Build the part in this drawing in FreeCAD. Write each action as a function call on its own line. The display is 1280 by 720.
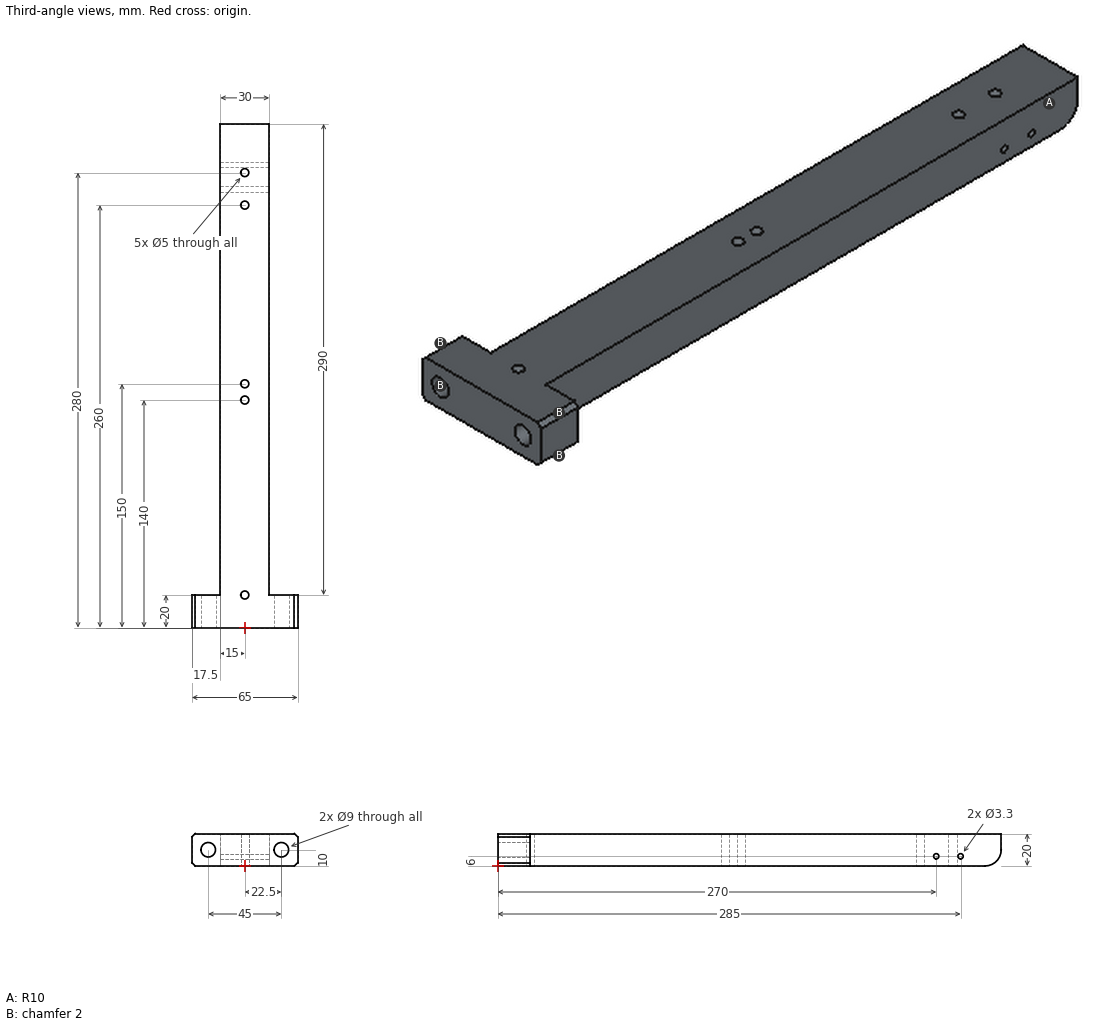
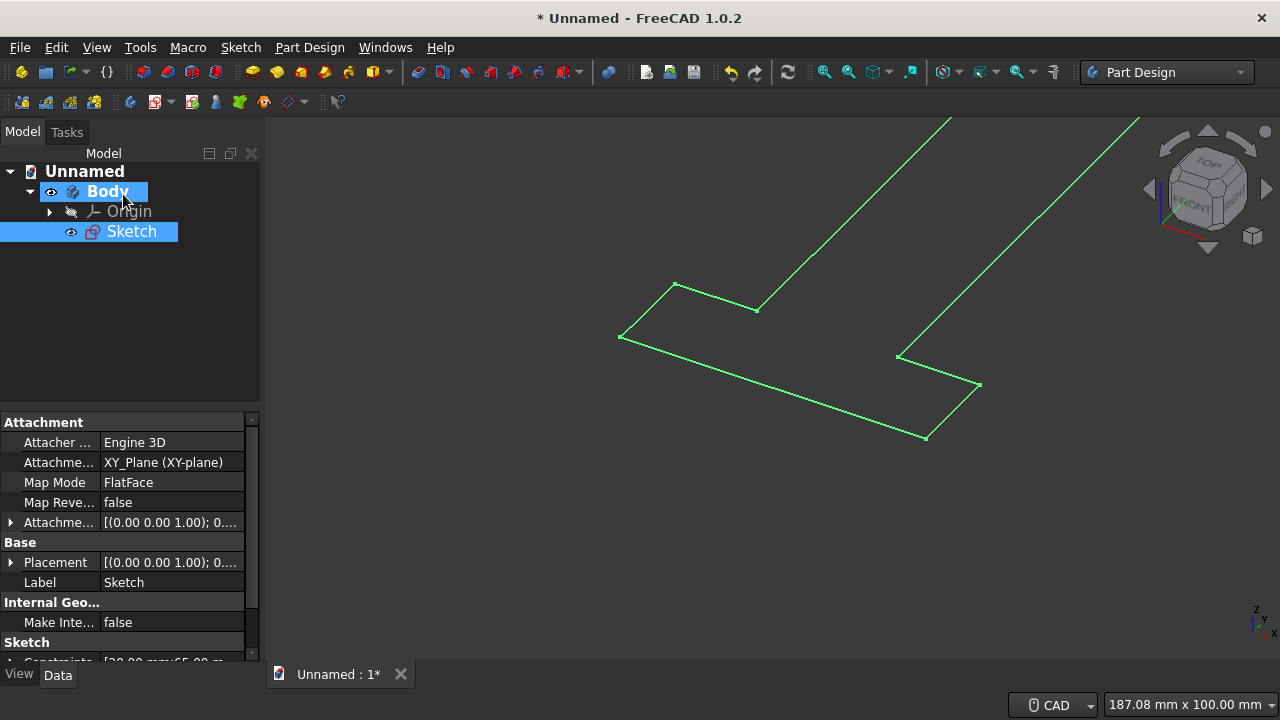
click(254, 72)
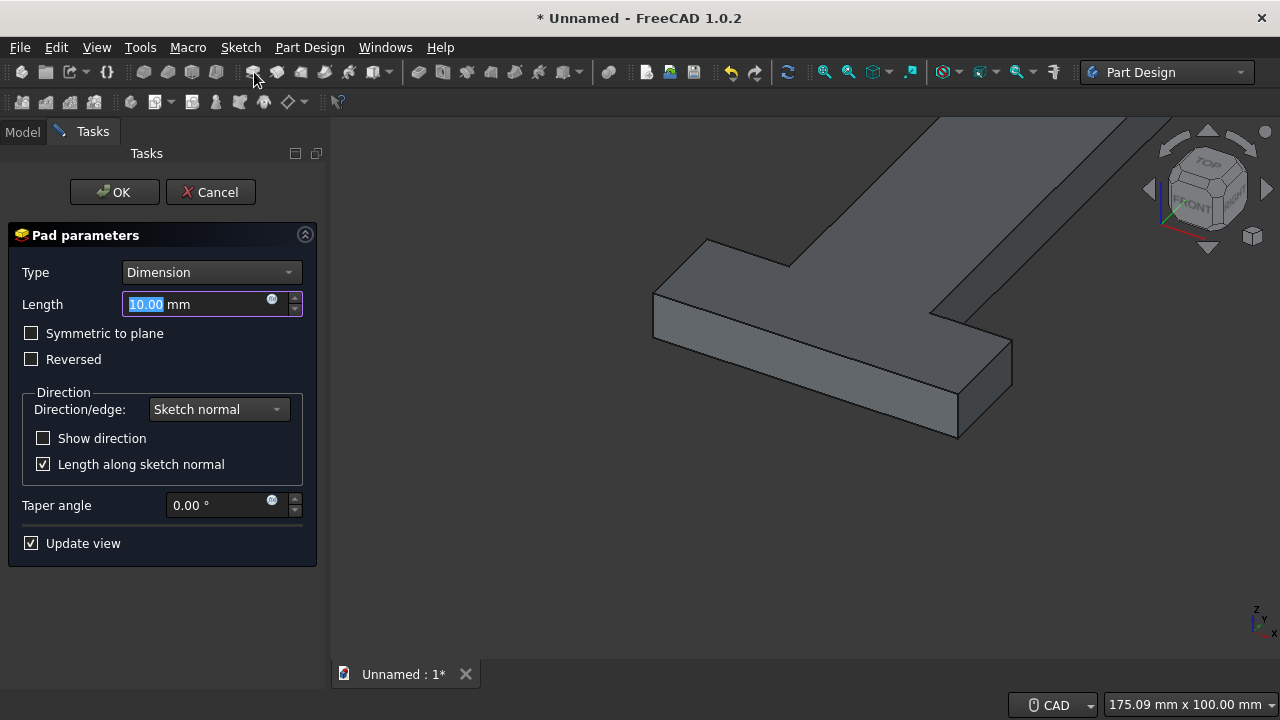
text(20)
key(Tab)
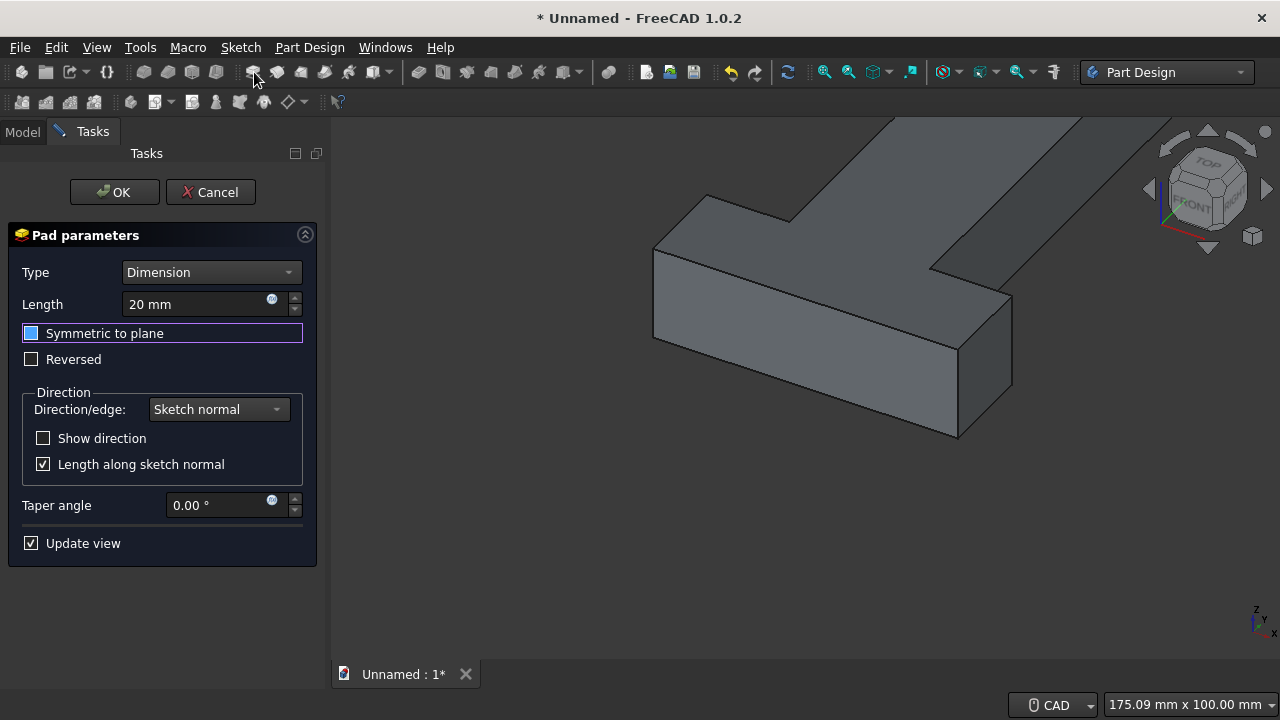
click(115, 192)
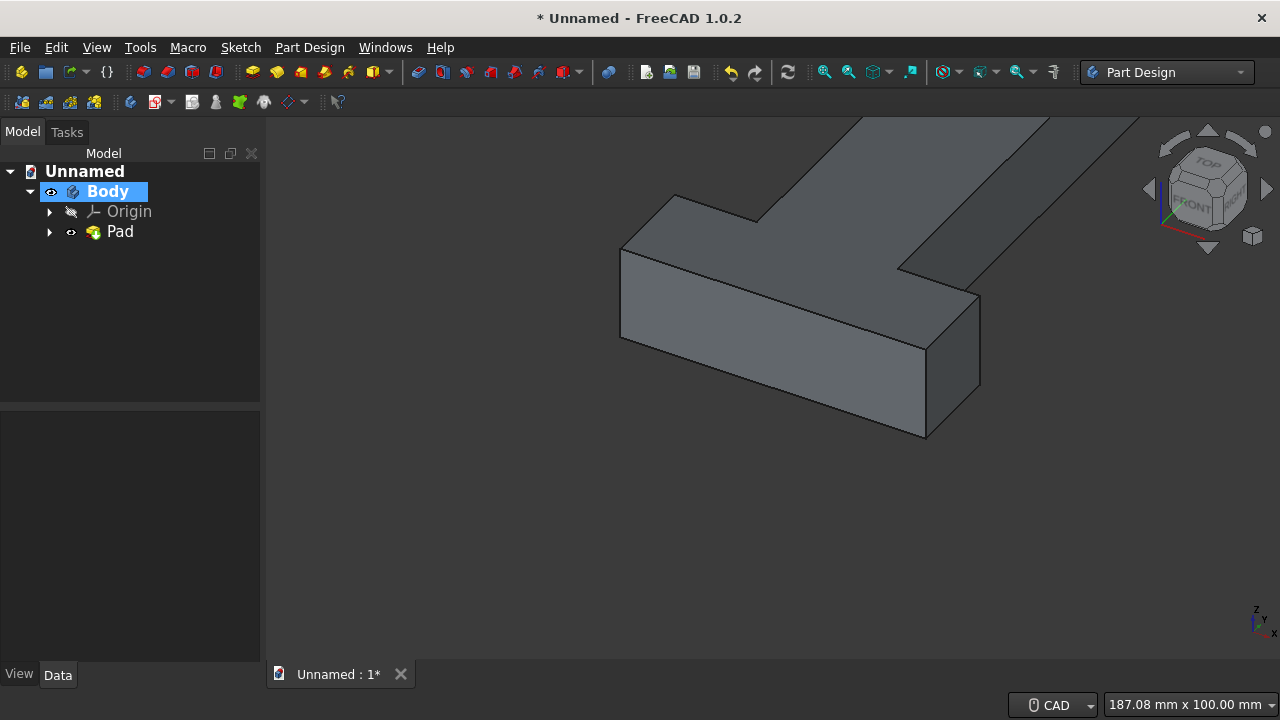
click(826, 72)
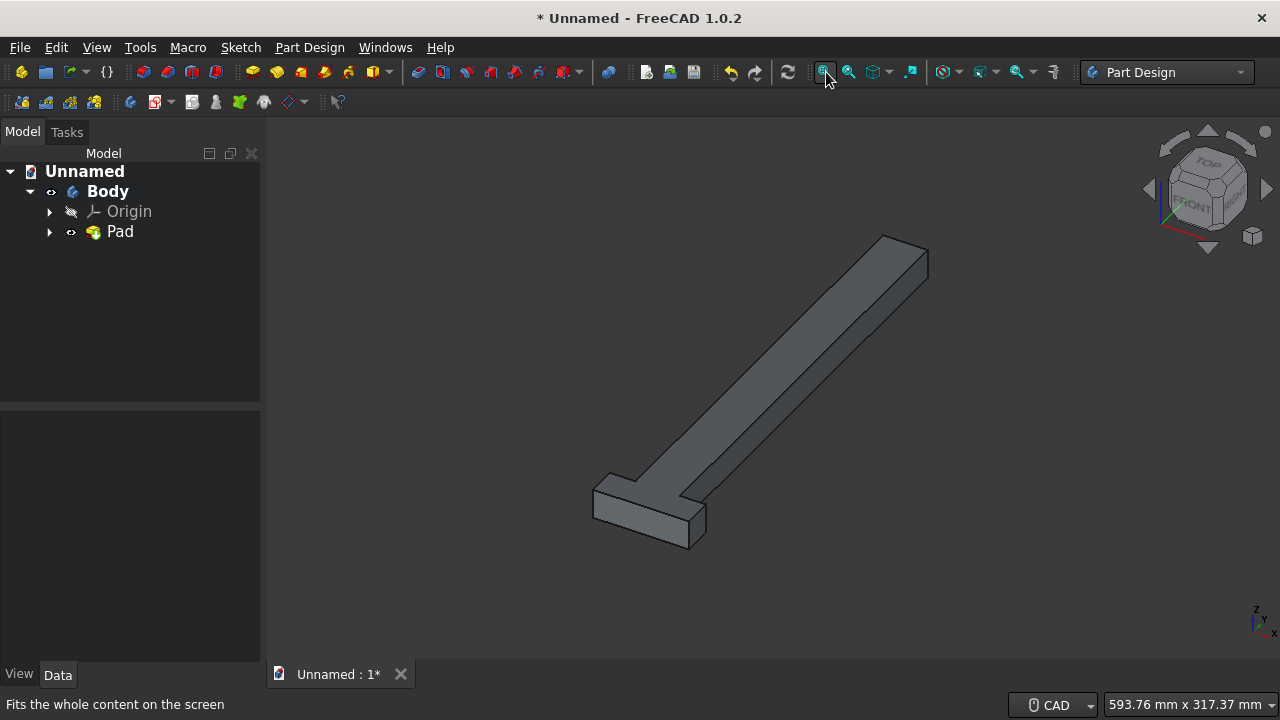
key(4)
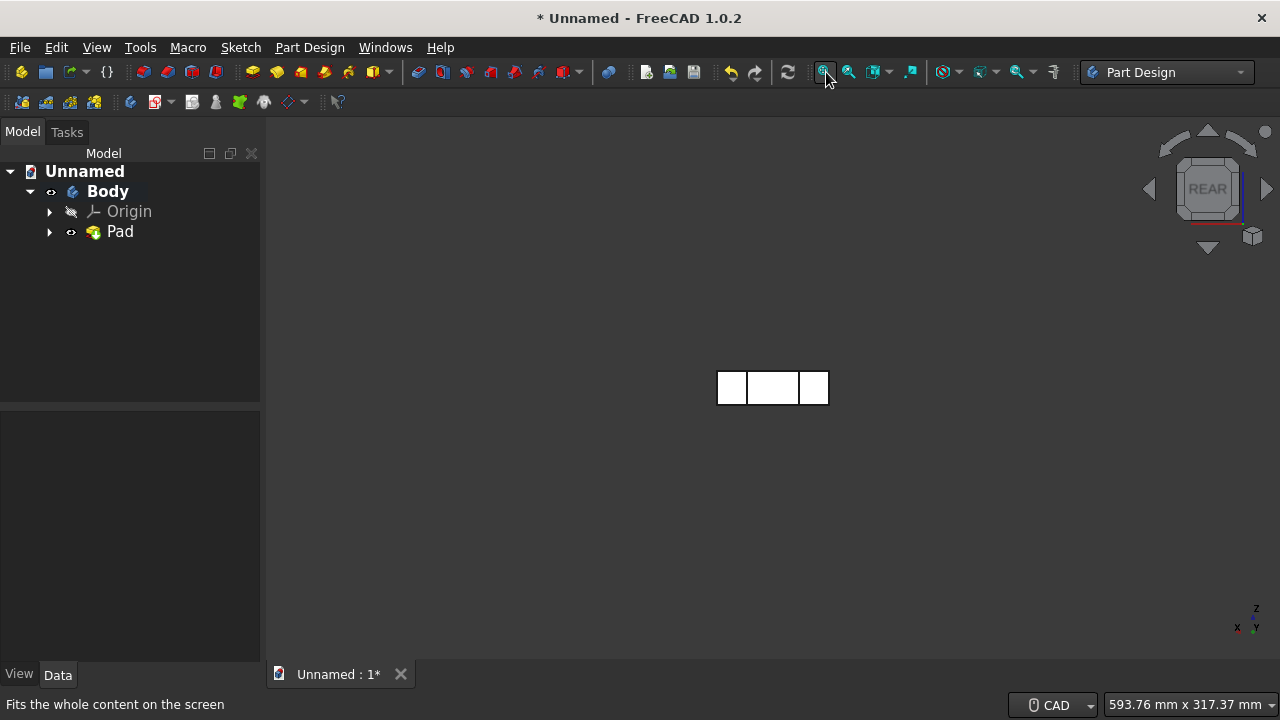
click(826, 72)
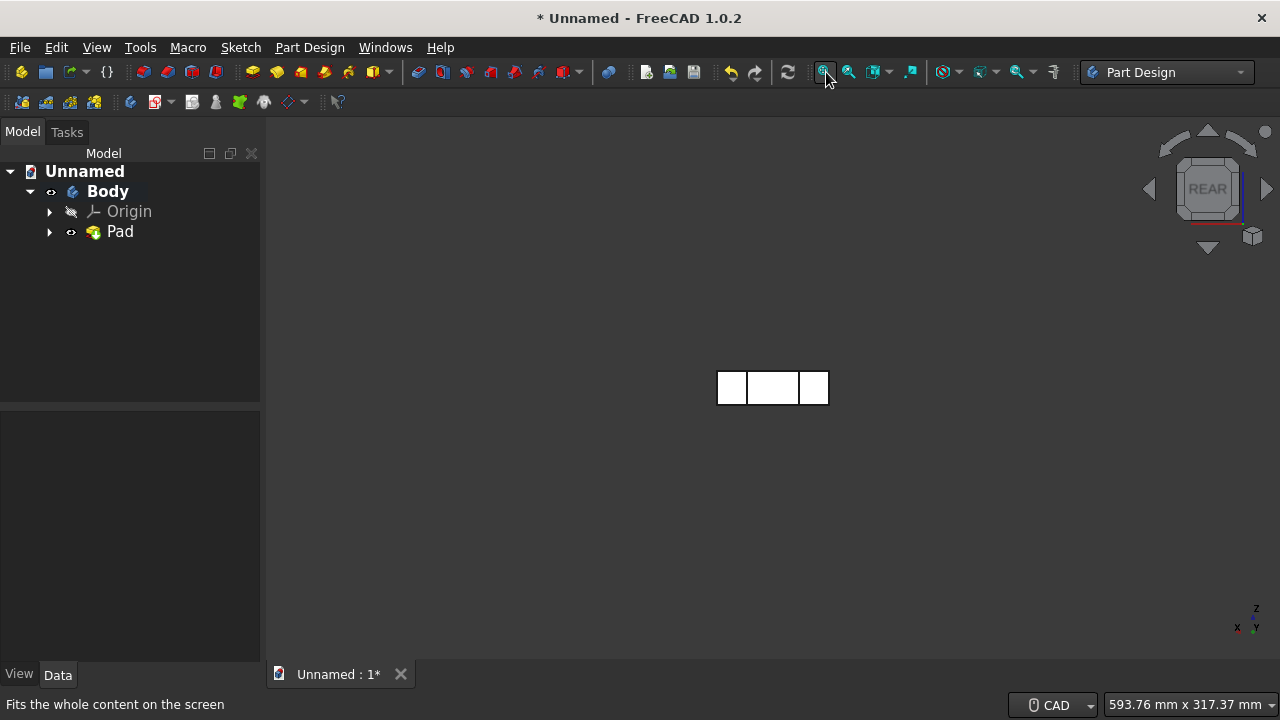
click(732, 387)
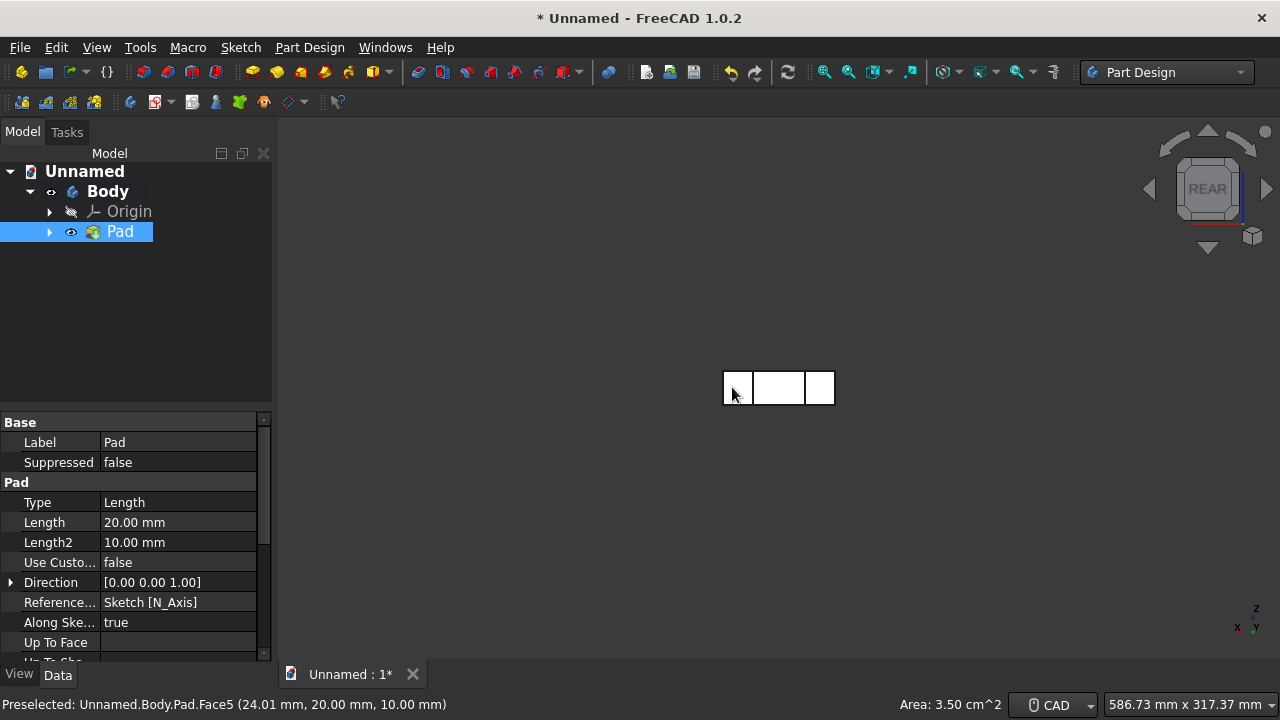
click(156, 102)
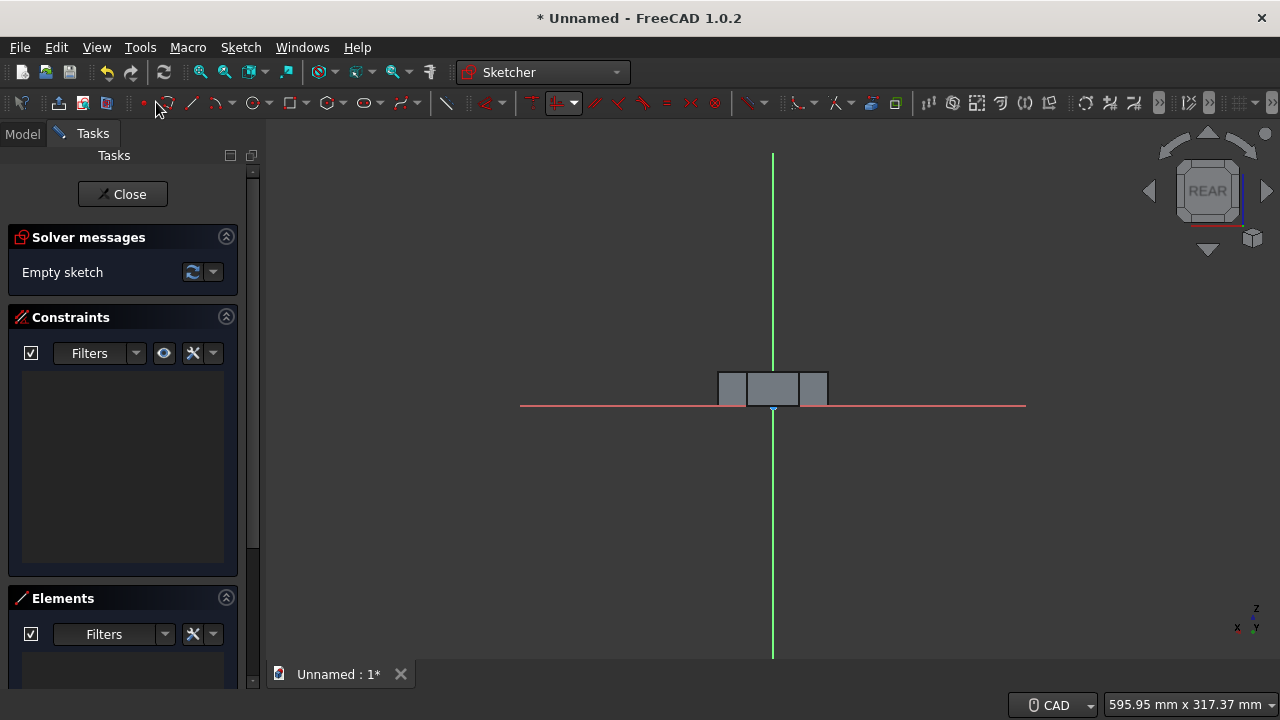
click(108, 104)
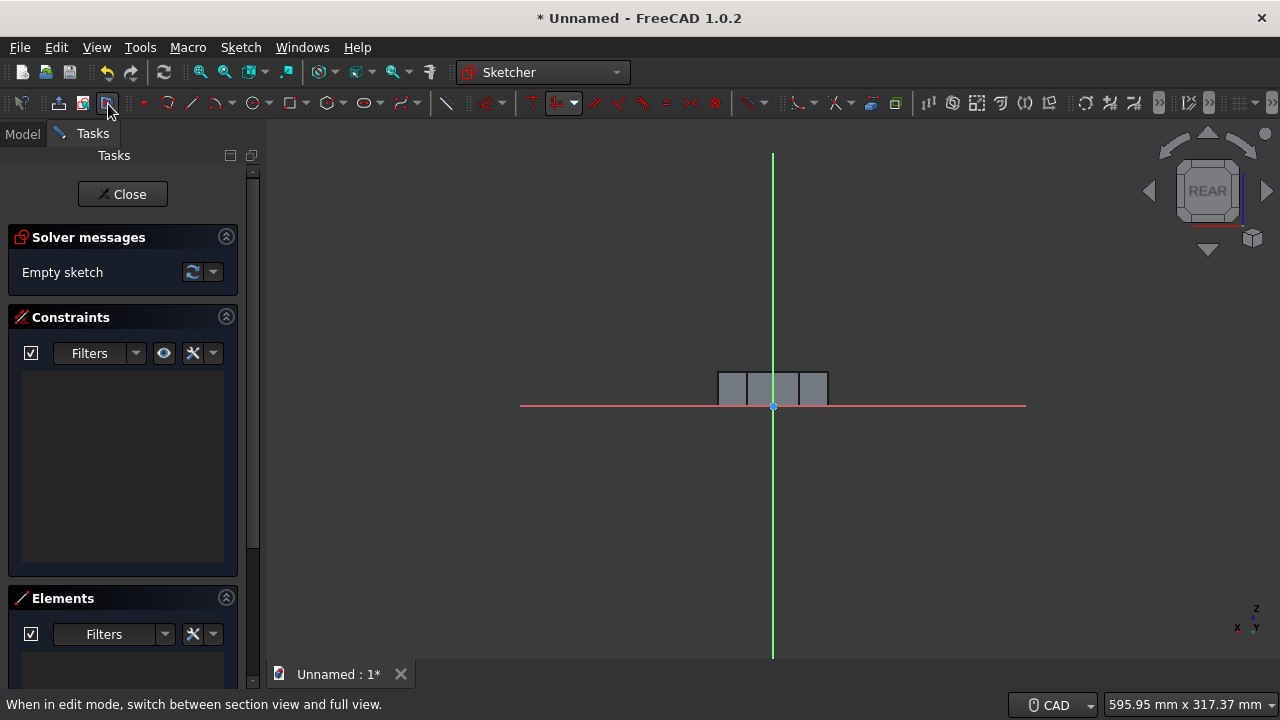
scroll(787, 395, up, 9)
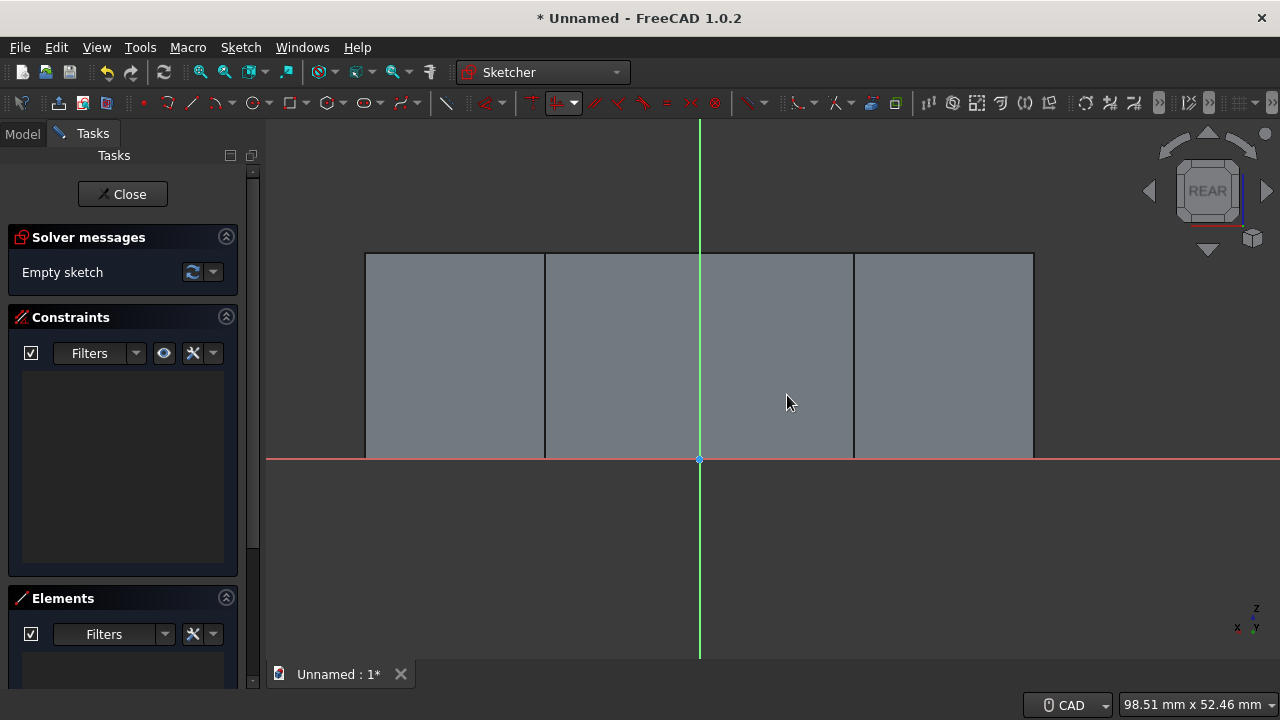
key(g)
key(c)